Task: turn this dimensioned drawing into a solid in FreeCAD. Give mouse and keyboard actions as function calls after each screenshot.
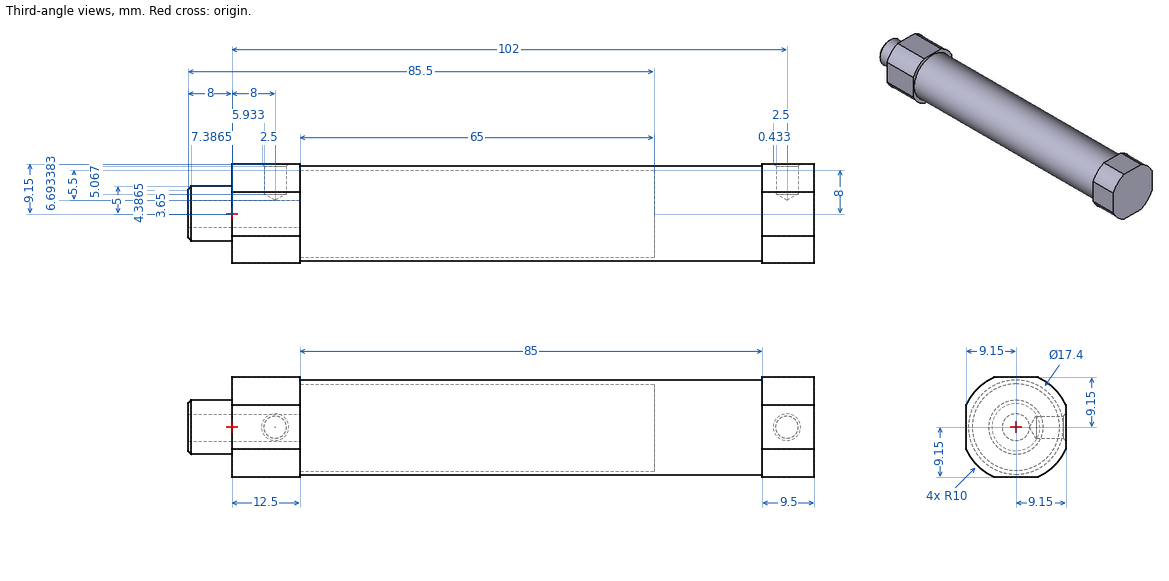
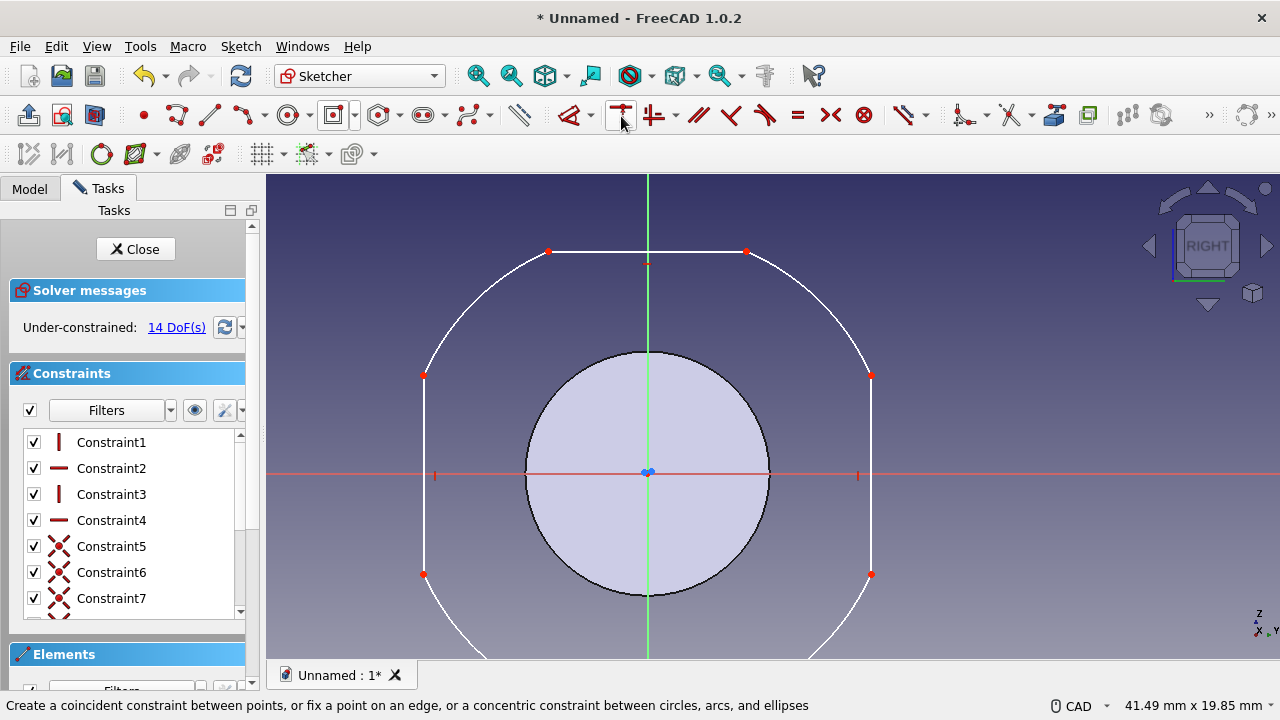
click(451, 621)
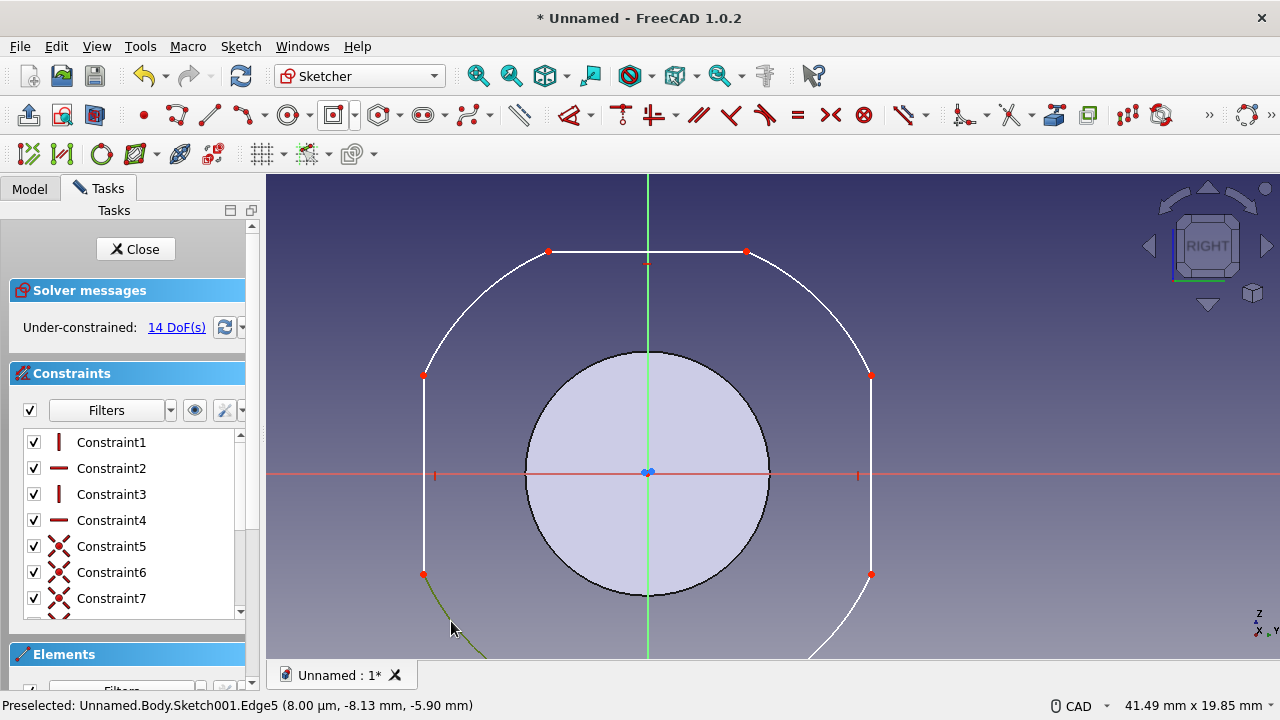
click(844, 329)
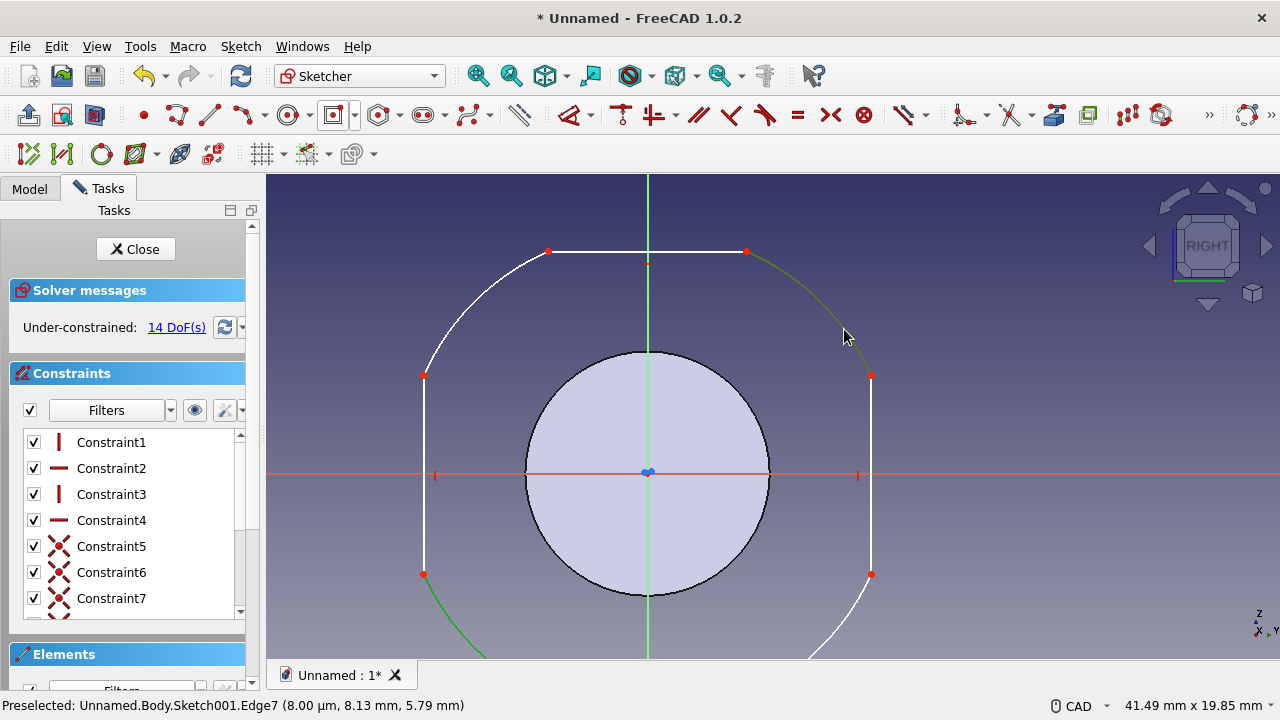
click(621, 116)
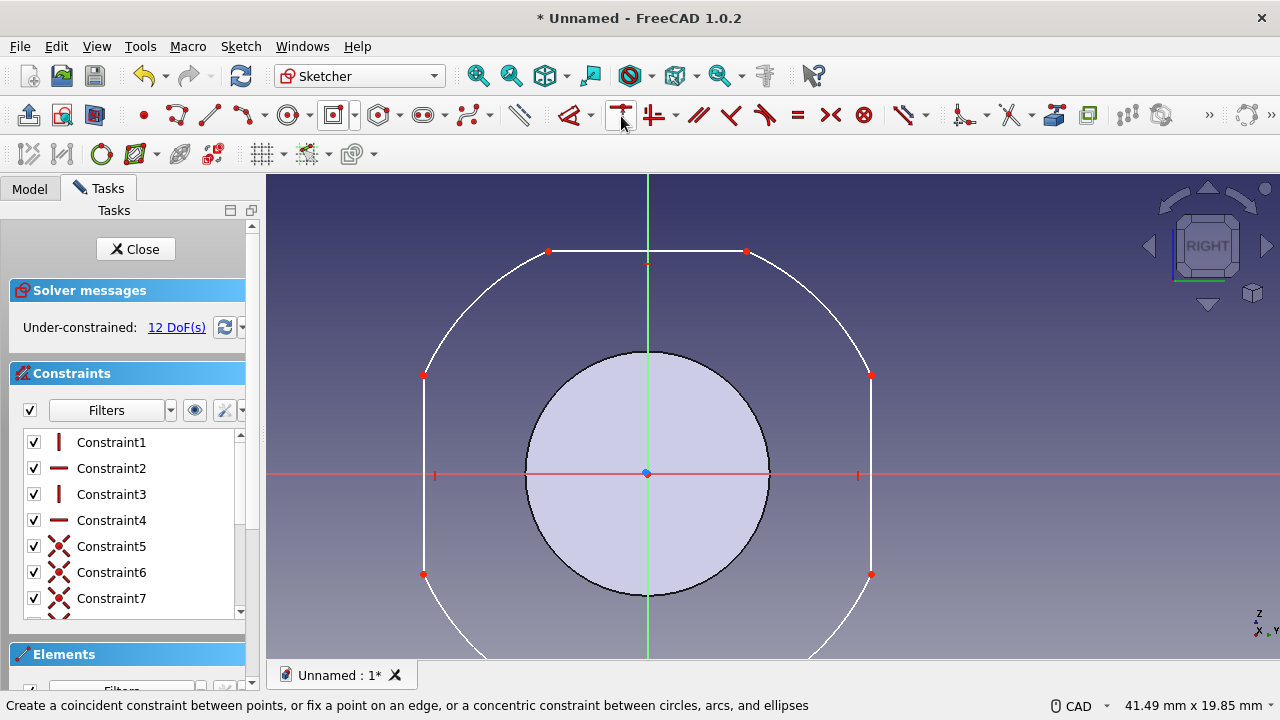
click(451, 621)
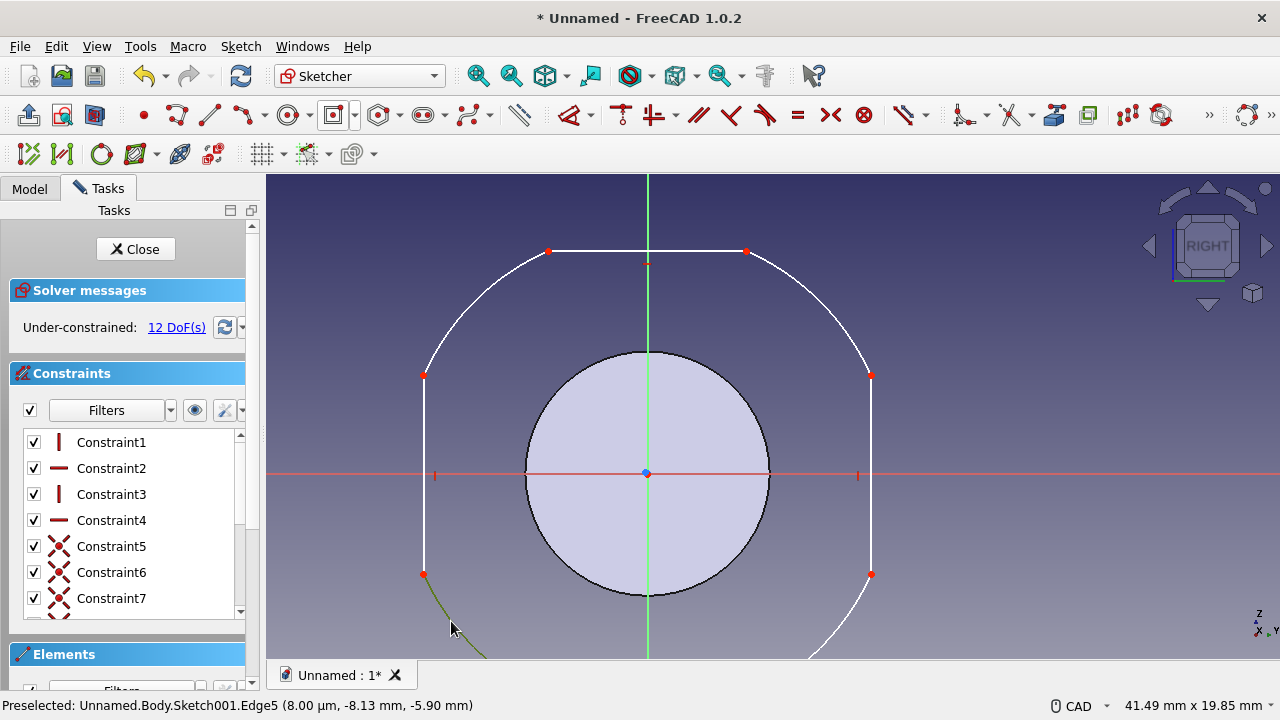
click(502, 278)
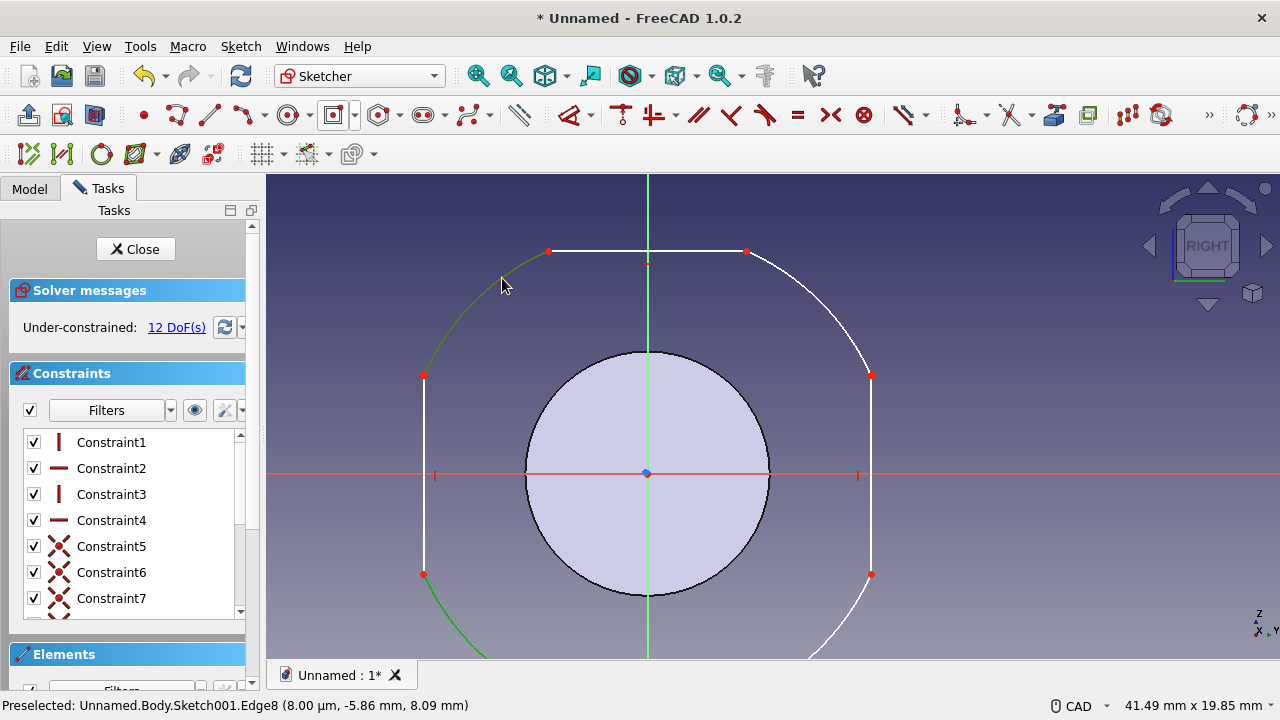
click(621, 116)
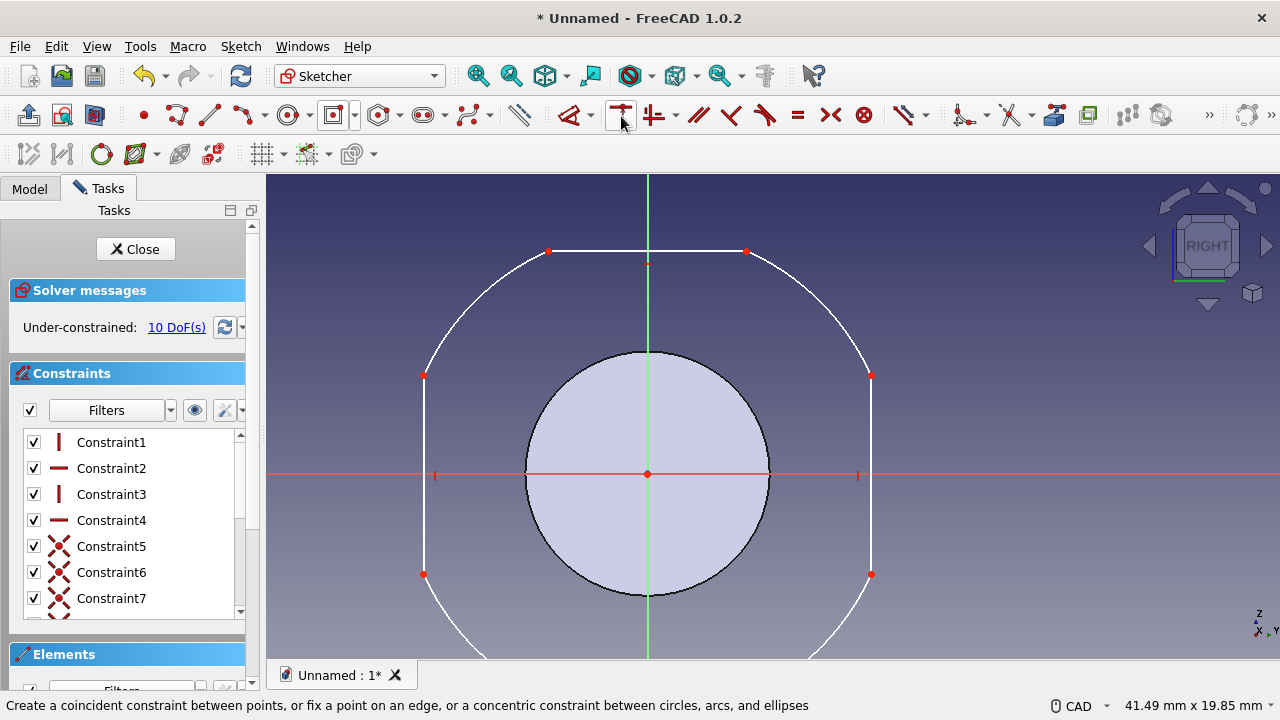
drag(637, 464, 658, 484)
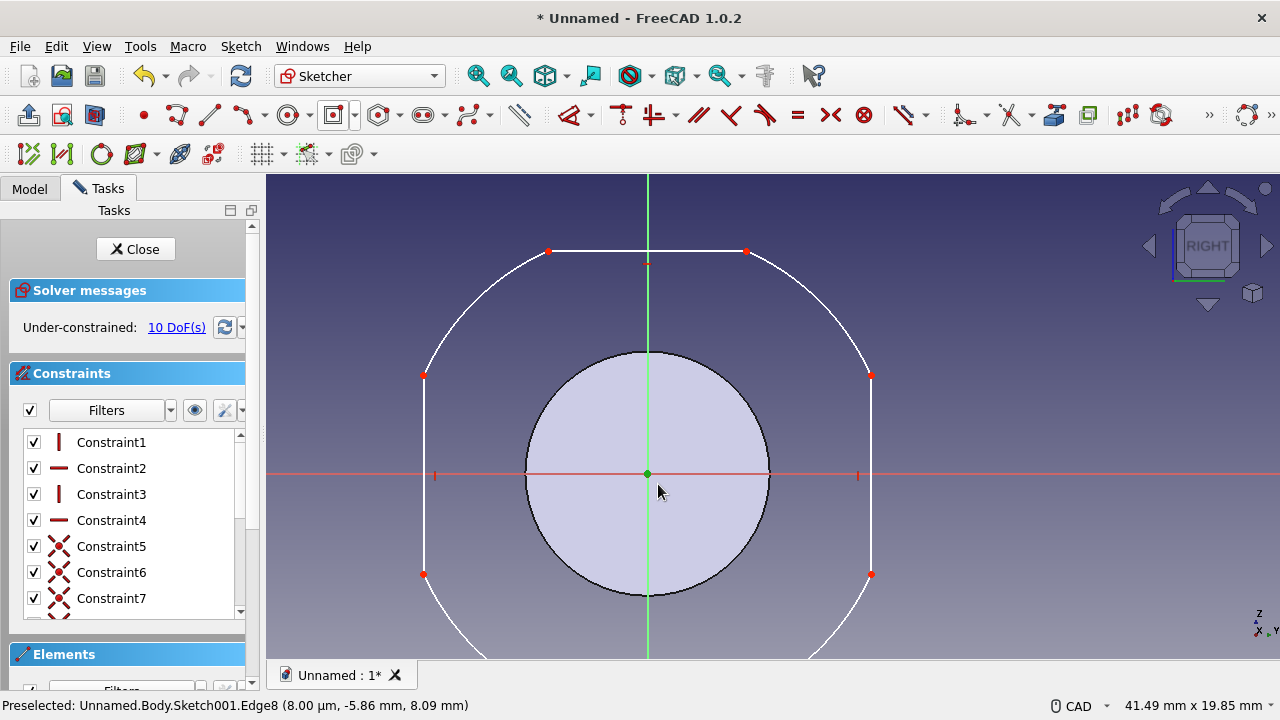
click(621, 116)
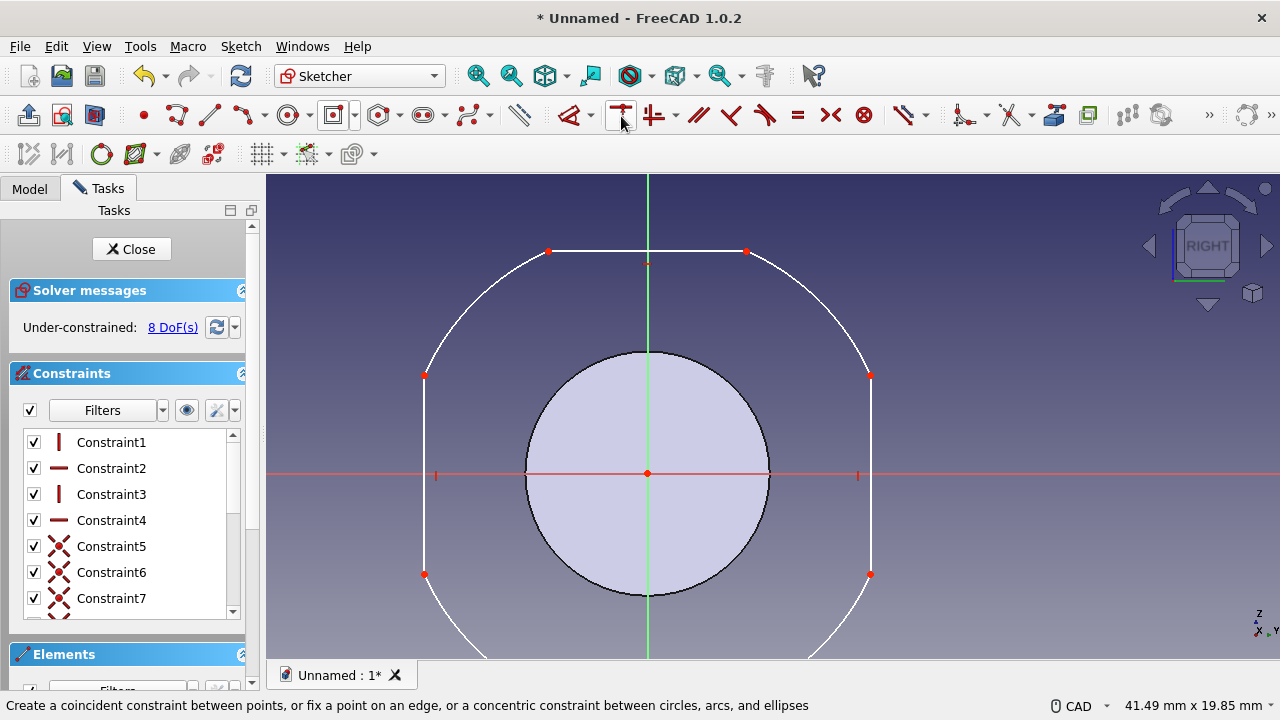
click(451, 620)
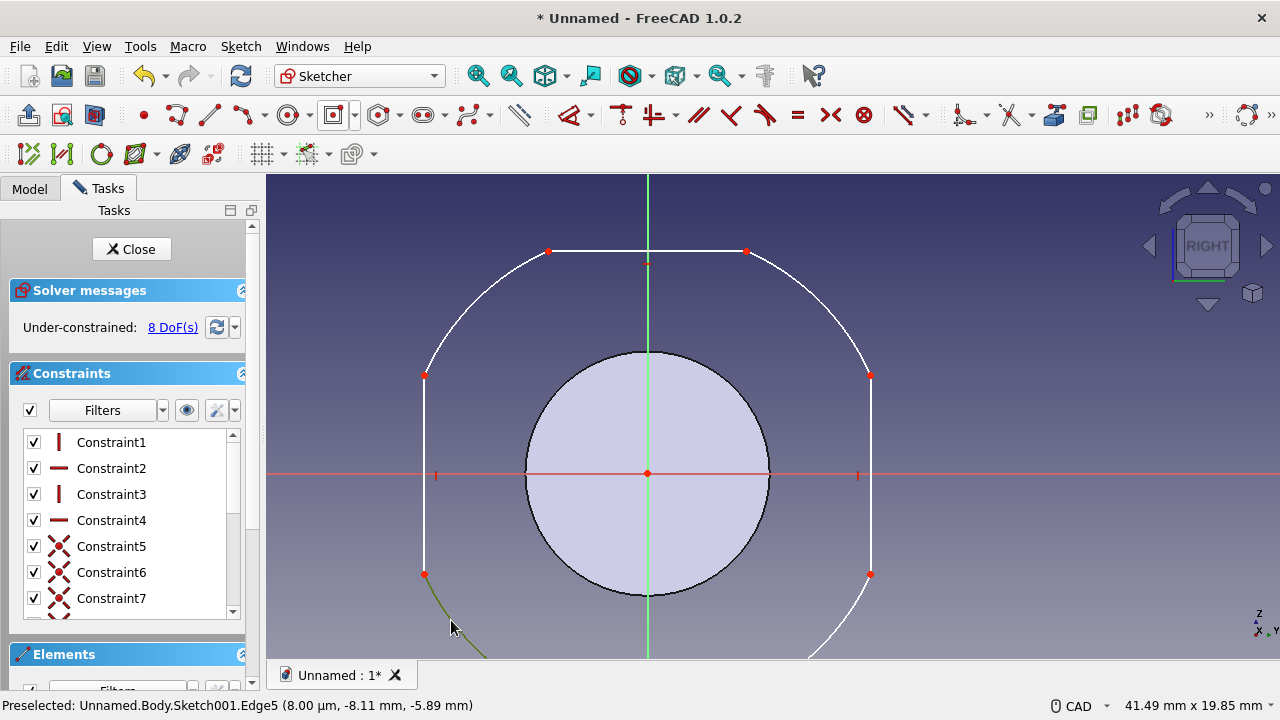
click(844, 621)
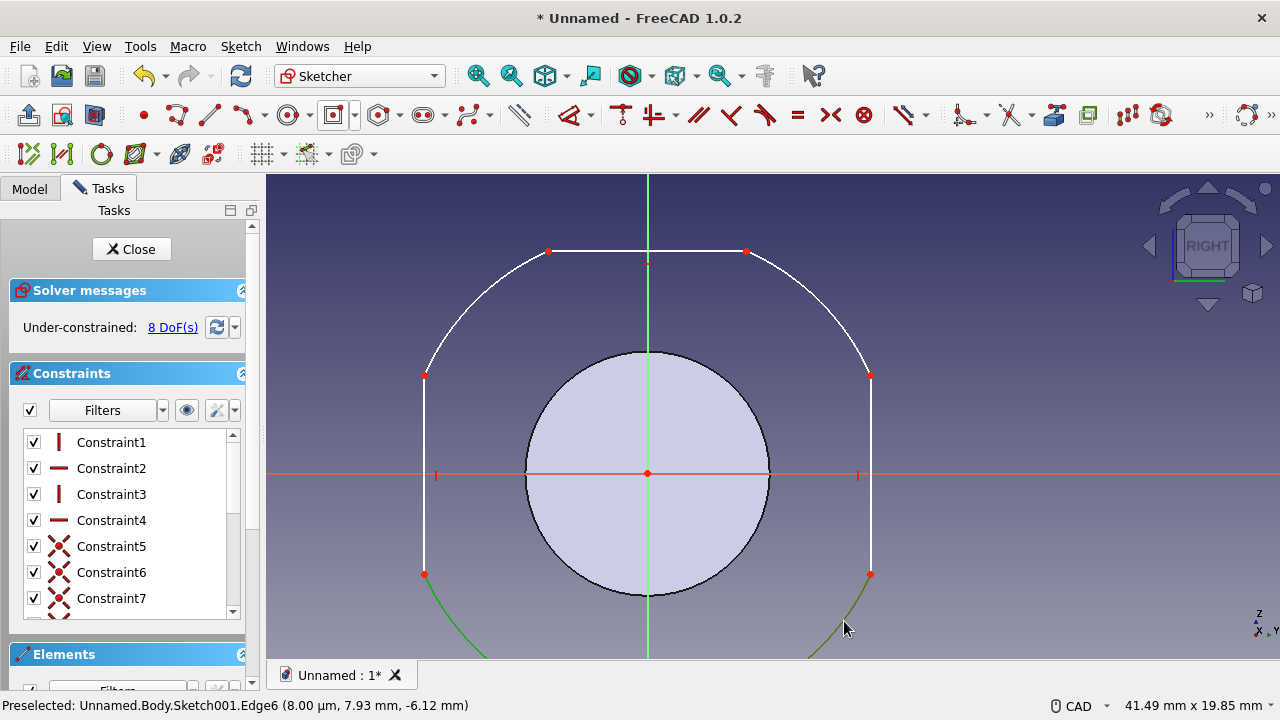
click(844, 329)